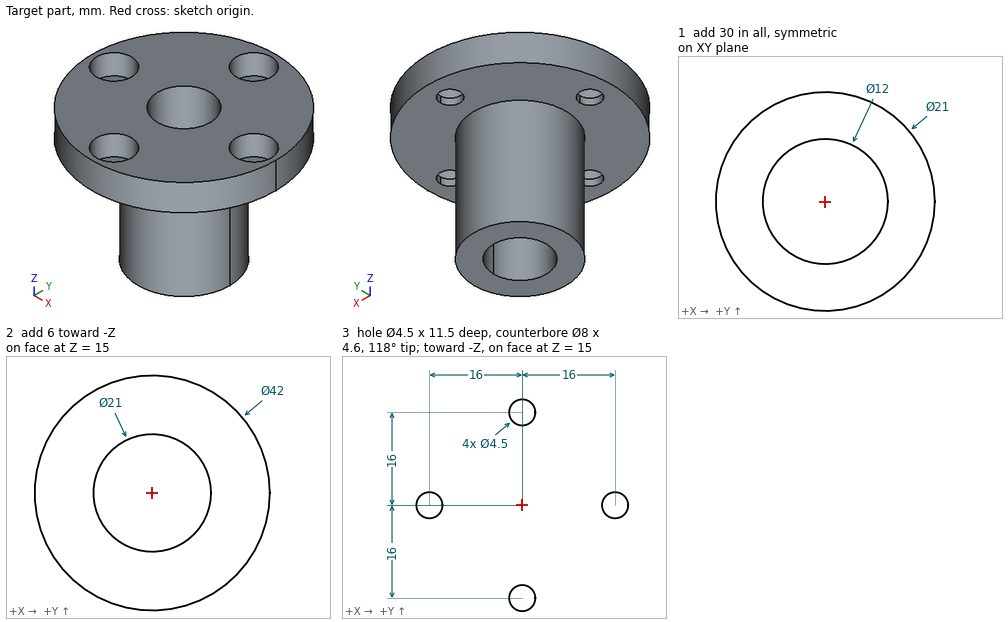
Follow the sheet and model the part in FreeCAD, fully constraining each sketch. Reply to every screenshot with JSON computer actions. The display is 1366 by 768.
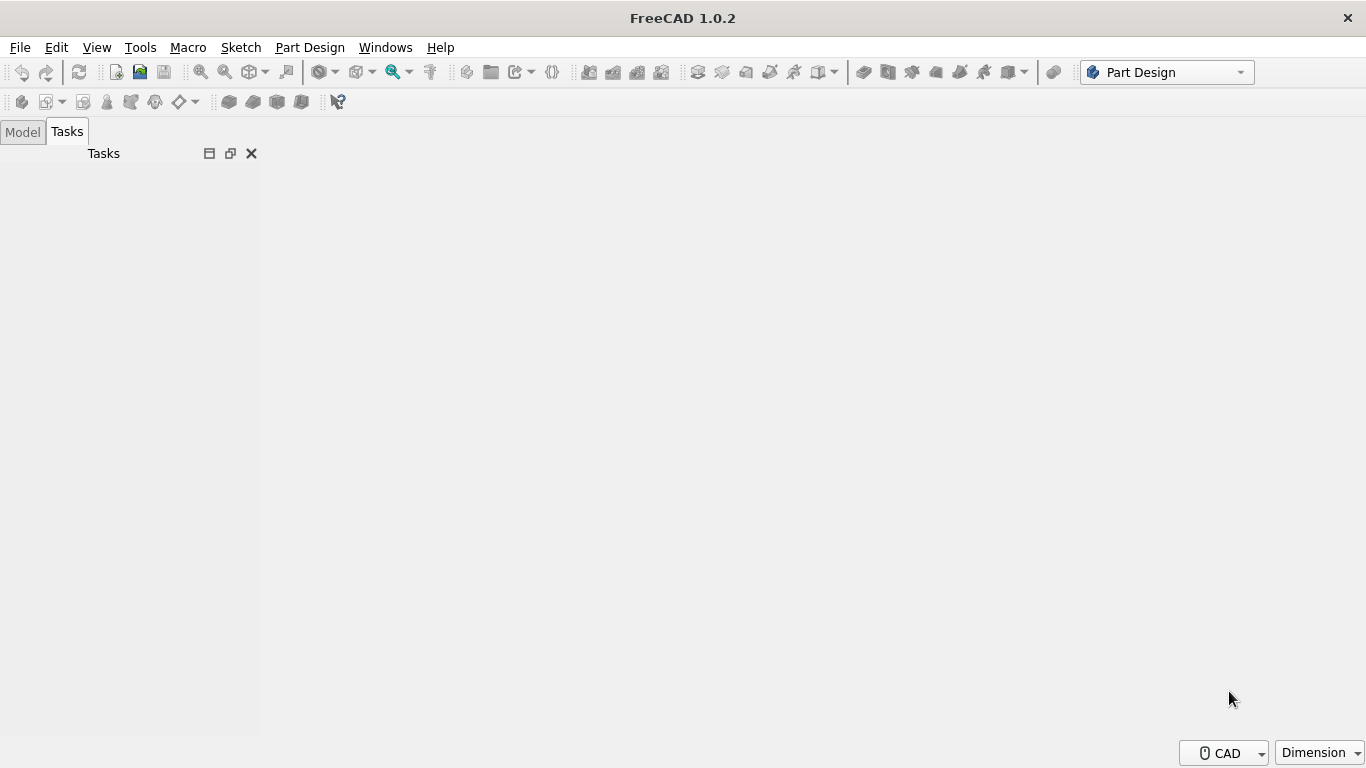
{"action": "left_click", "coordinate": [116, 72]}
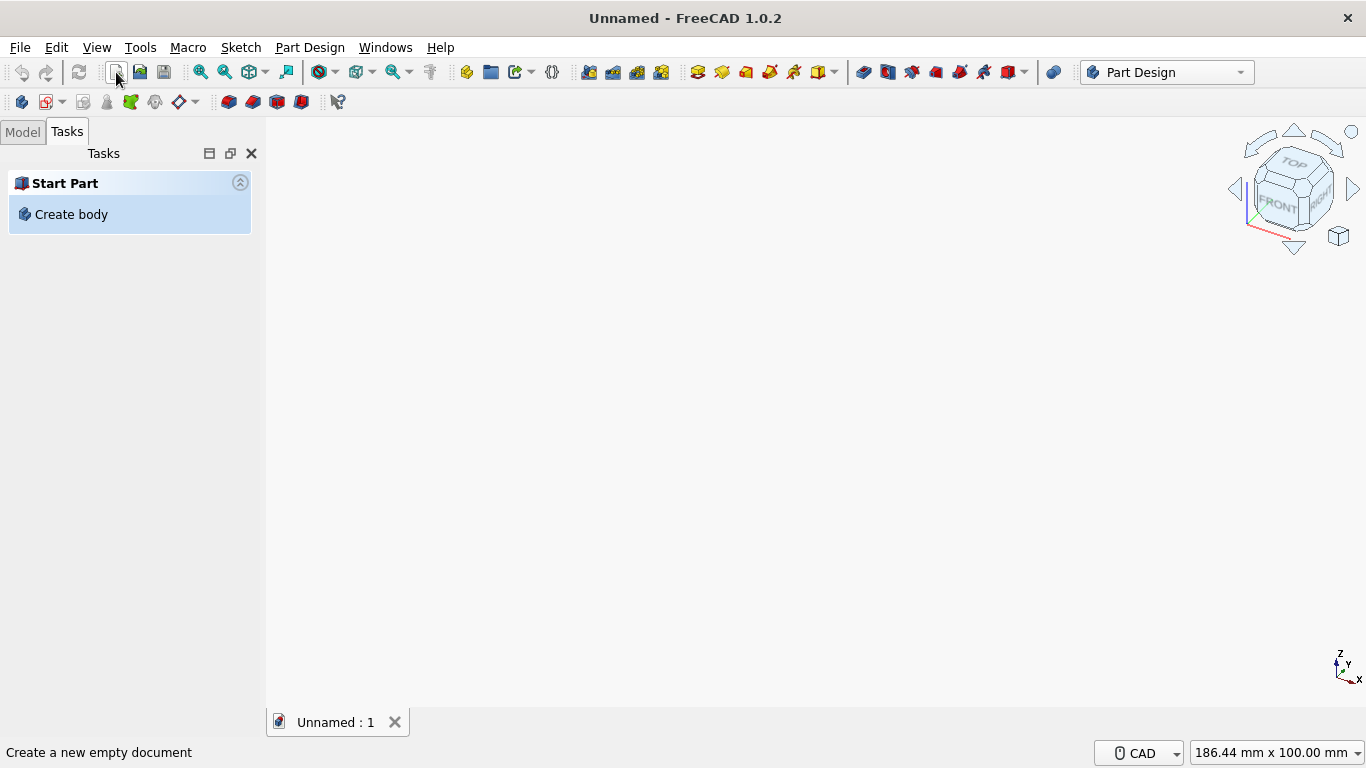
{"action": "left_click", "coordinate": [46, 102]}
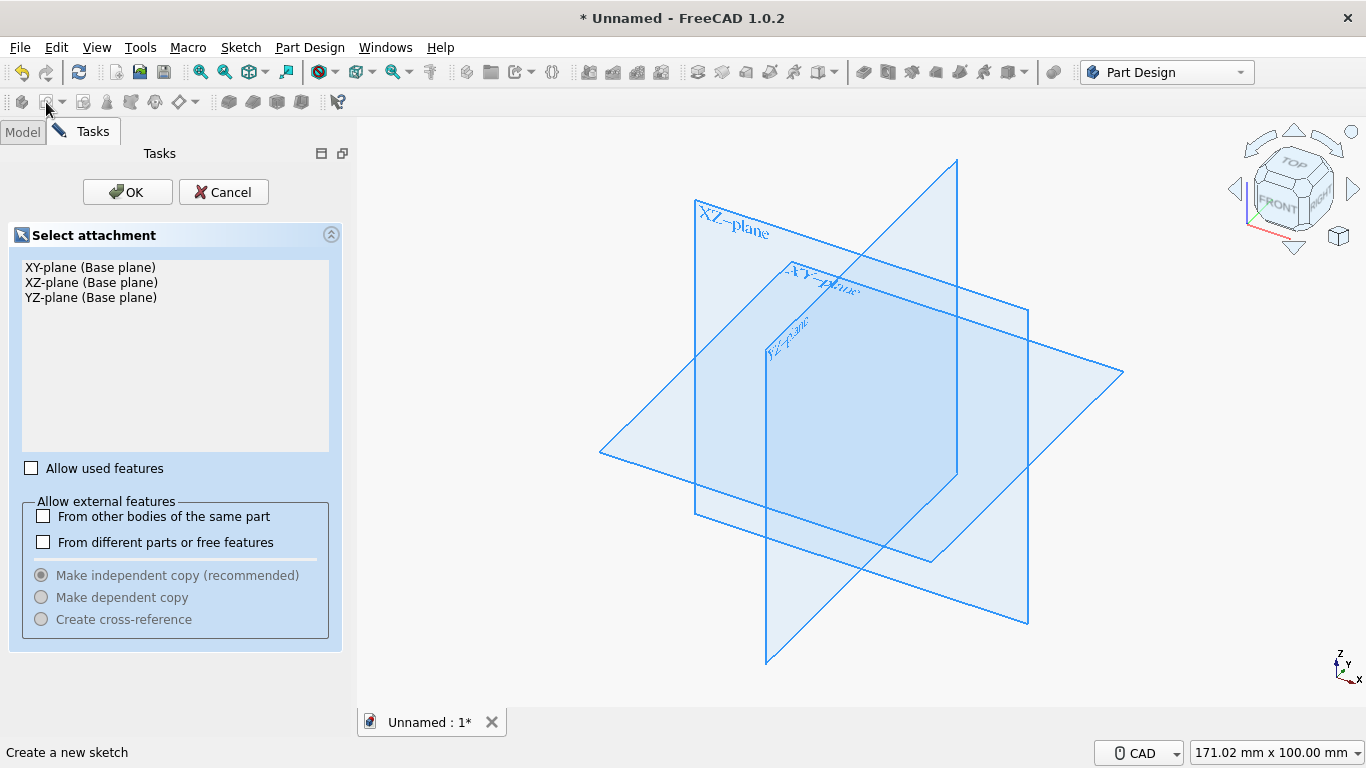
{"action": "left_click", "coordinate": [82, 268]}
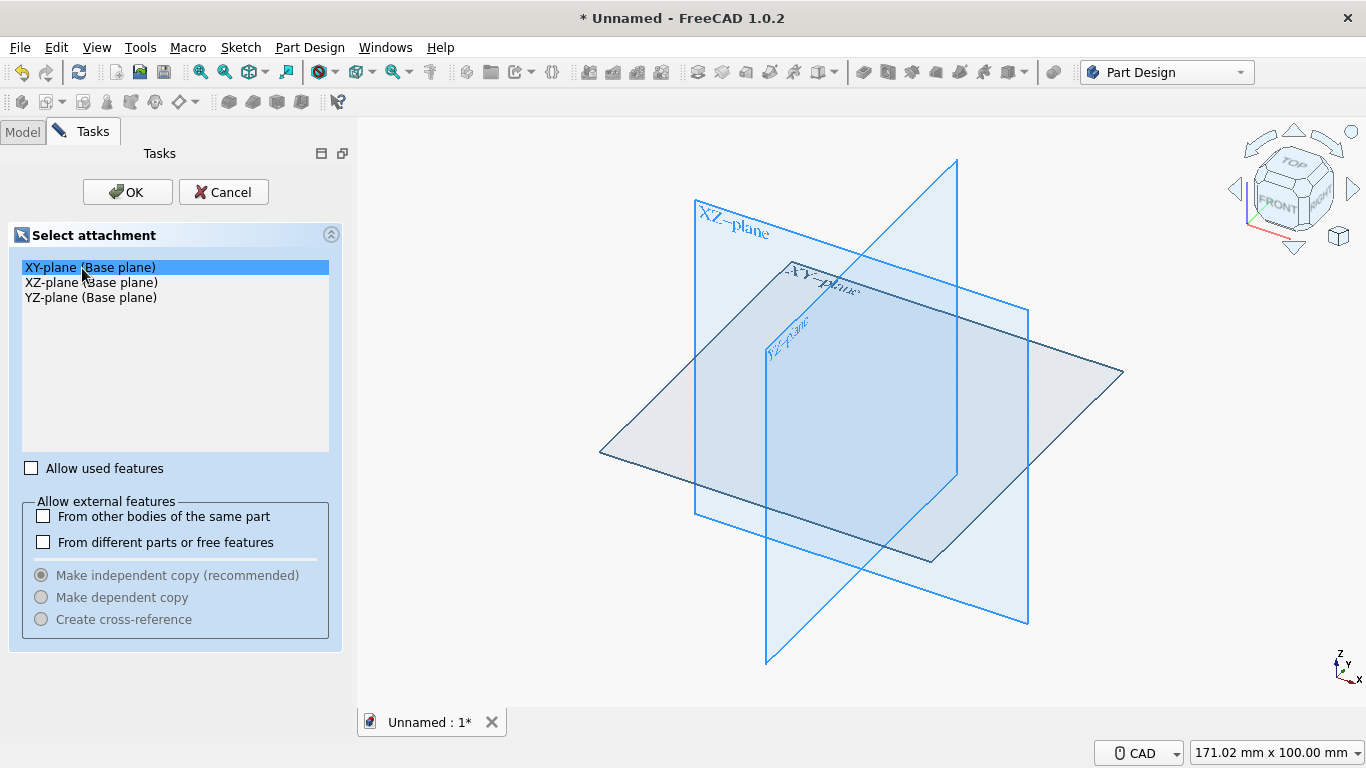
{"action": "left_click", "coordinate": [128, 192]}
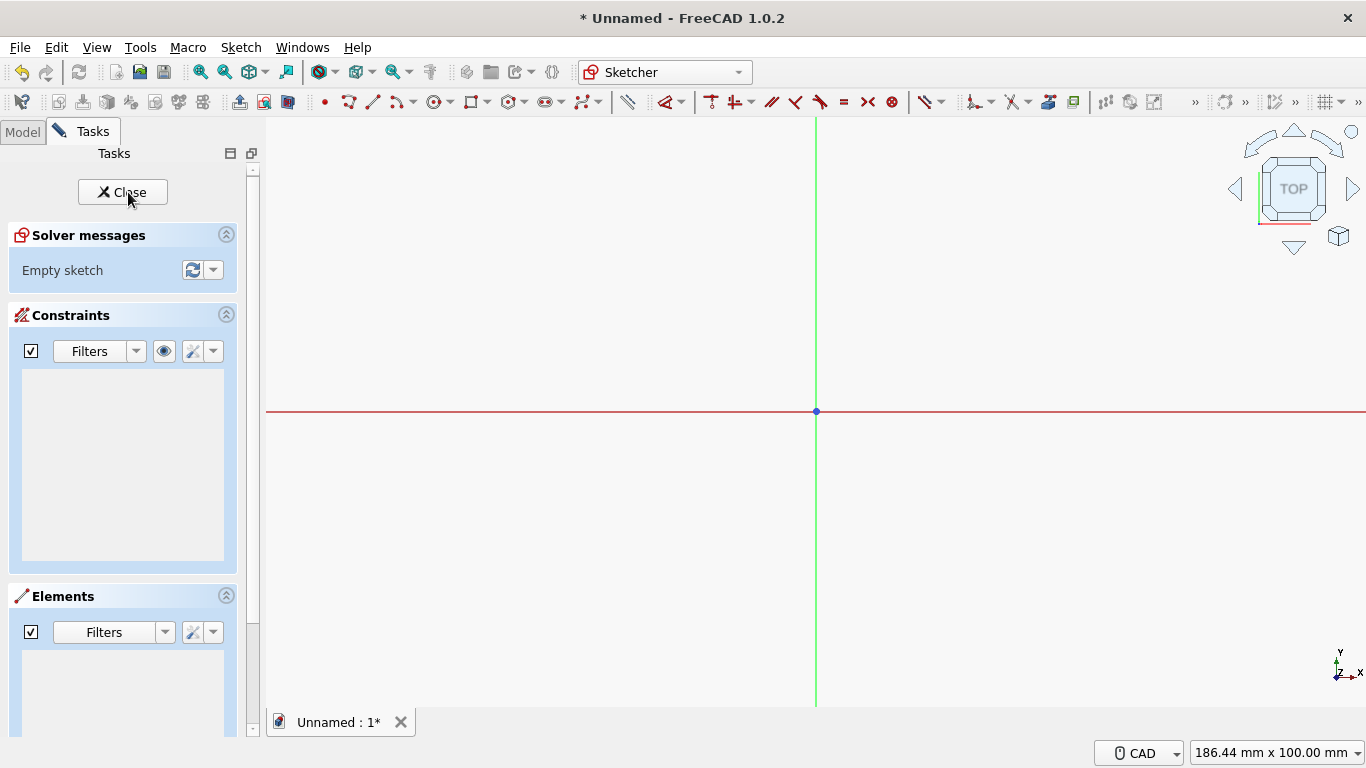
{"action": "scroll", "coordinate": [846, 412], "scroll_direction": "up", "scroll_amount": 6}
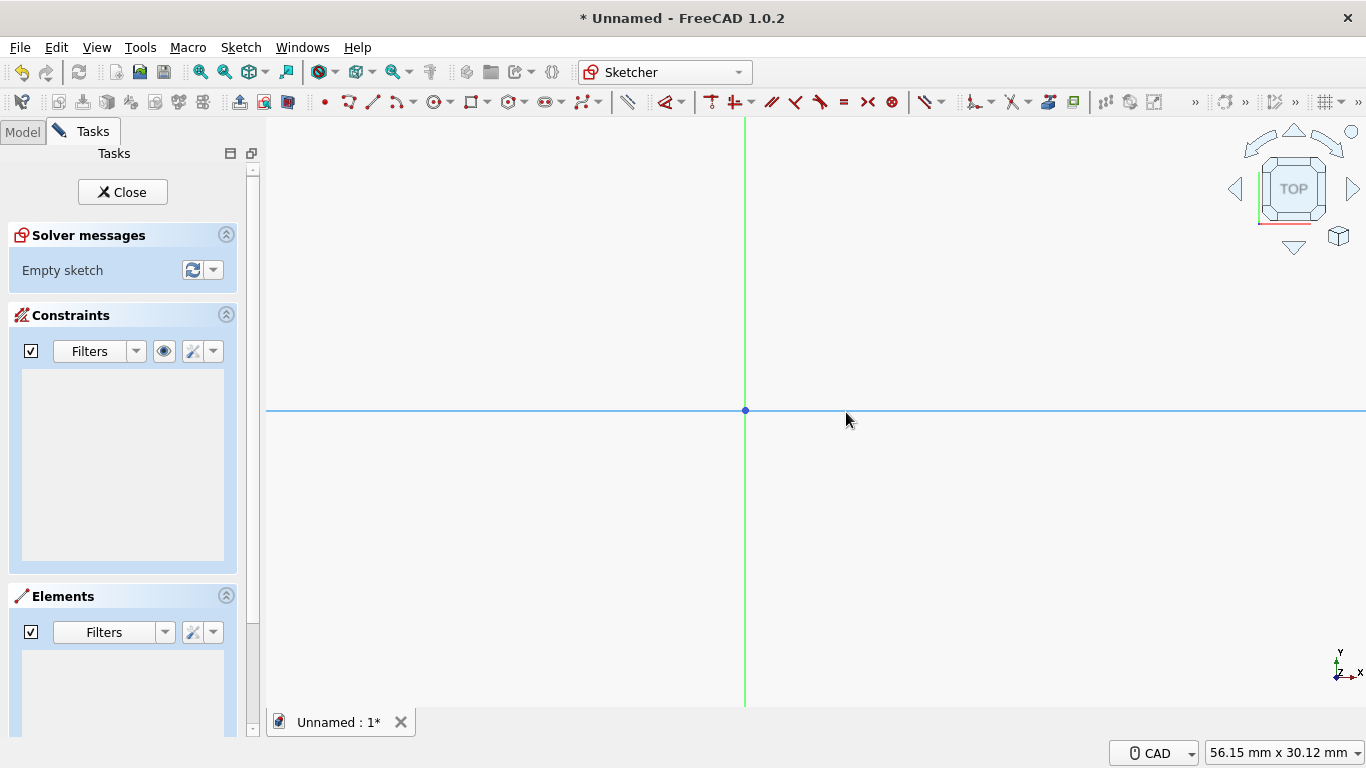
{"action": "left_click", "coordinate": [434, 102]}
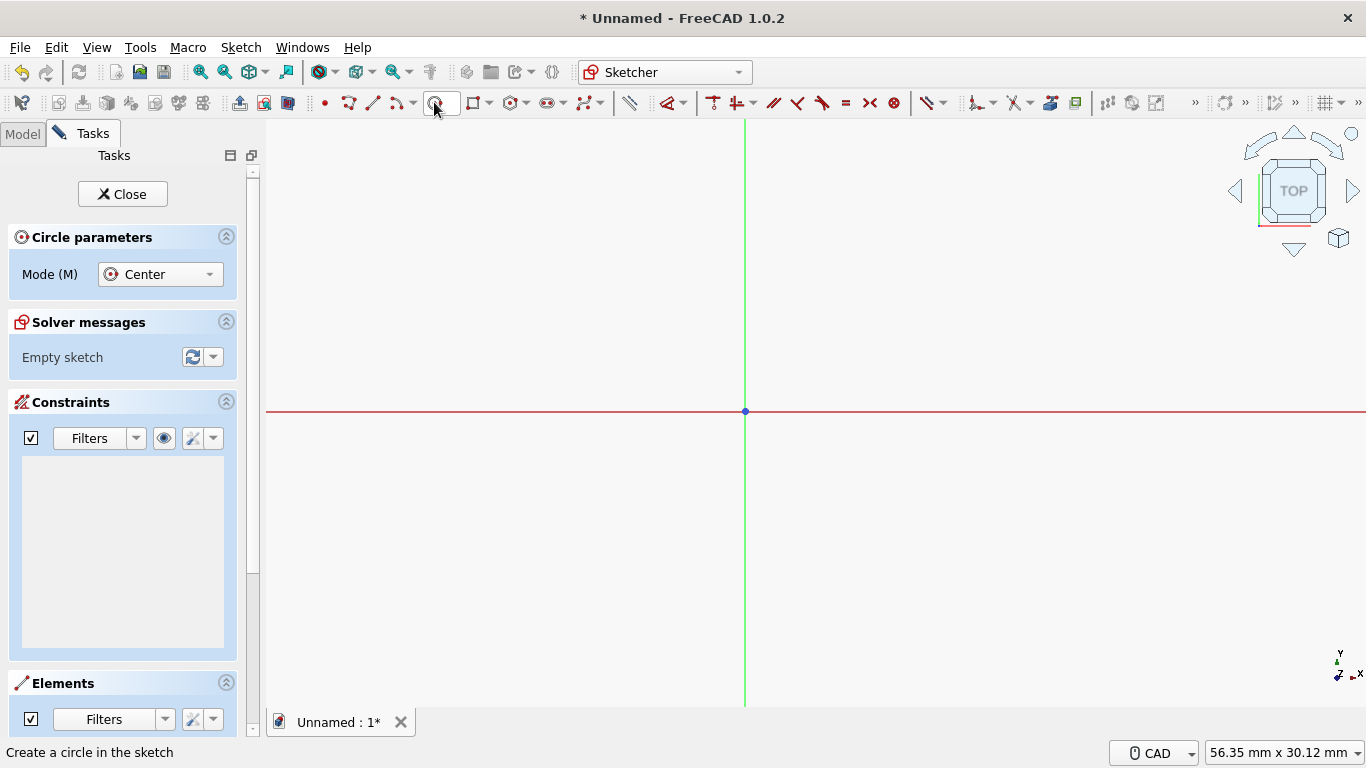
{"action": "left_click", "coordinate": [745, 412]}
{"action": "mouse_move", "coordinate": [890, 267]}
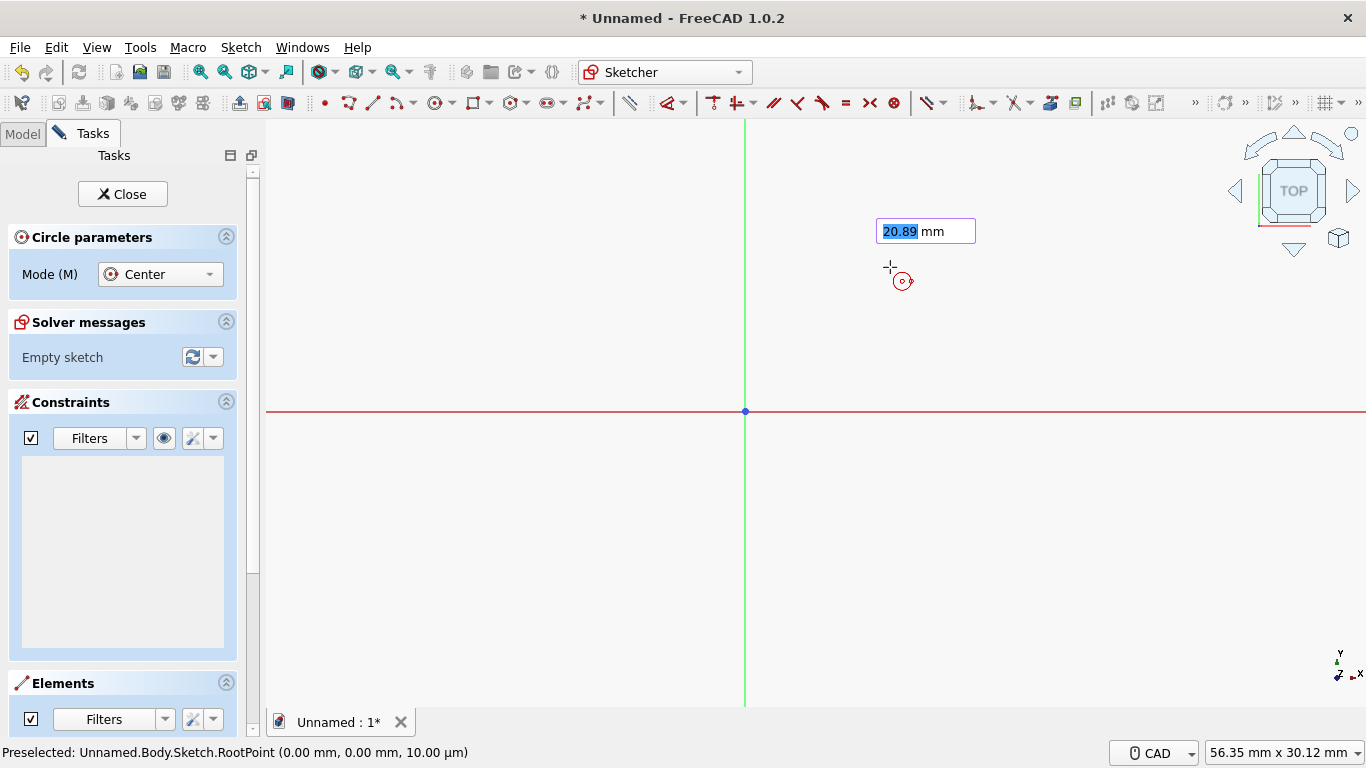
{"action": "type", "text": "21"}
{"action": "key", "text": "Return"}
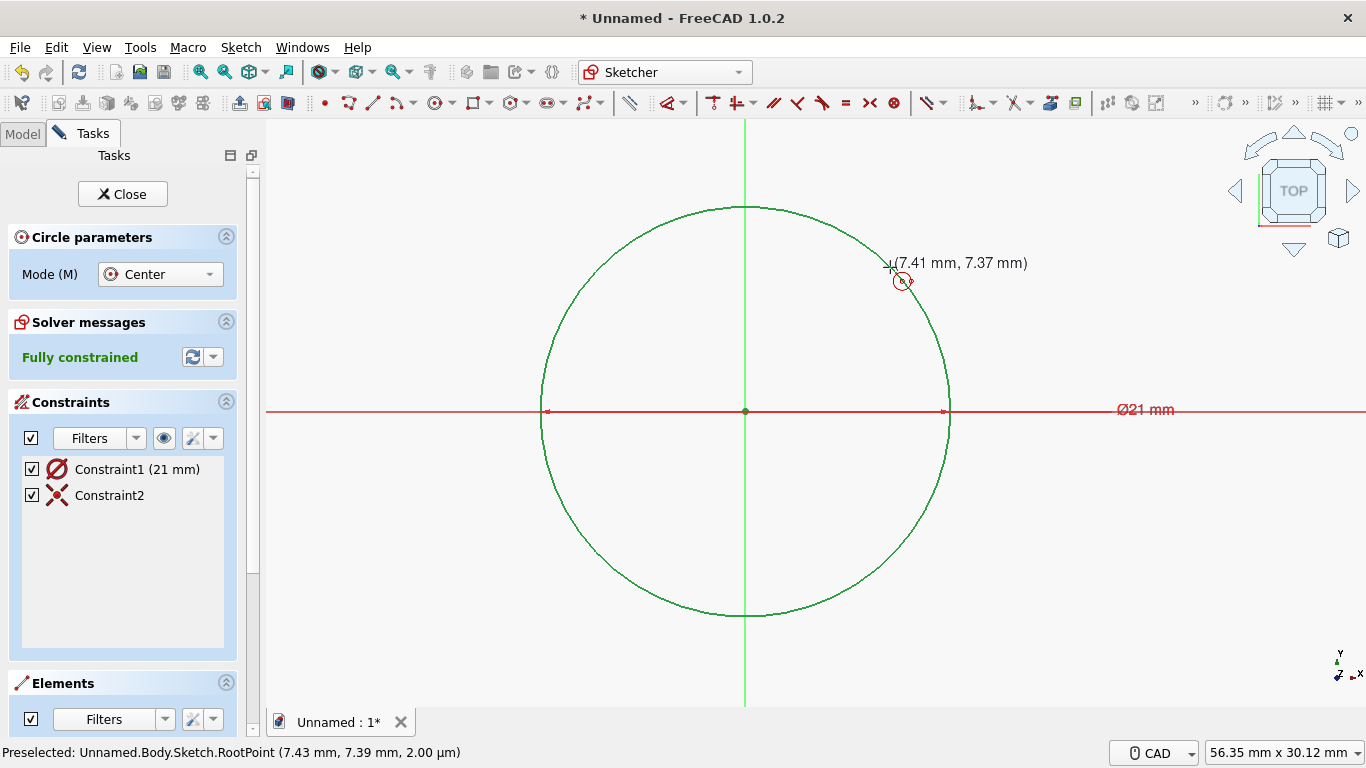
{"action": "left_click", "coordinate": [745, 412]}
{"action": "mouse_move", "coordinate": [828, 329]}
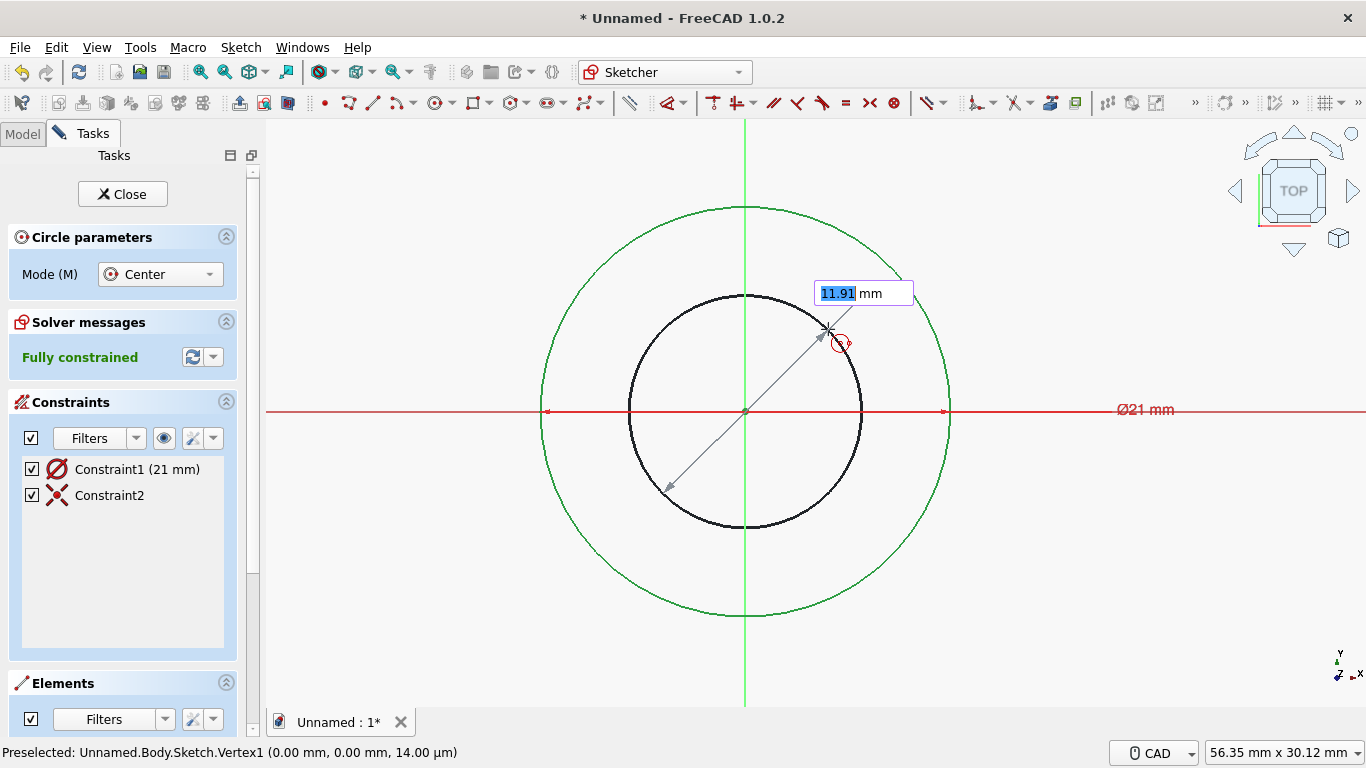
{"action": "type", "text": "12"}
{"action": "key", "text": "Return"}
{"action": "key", "text": "Escape"}